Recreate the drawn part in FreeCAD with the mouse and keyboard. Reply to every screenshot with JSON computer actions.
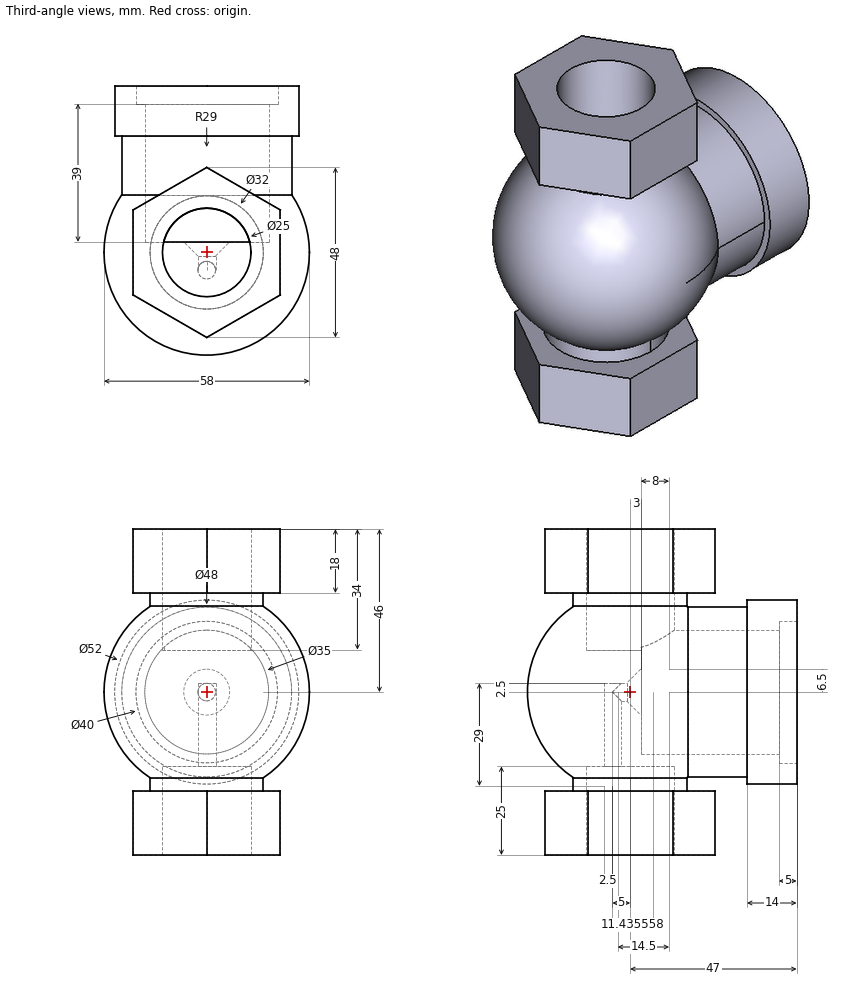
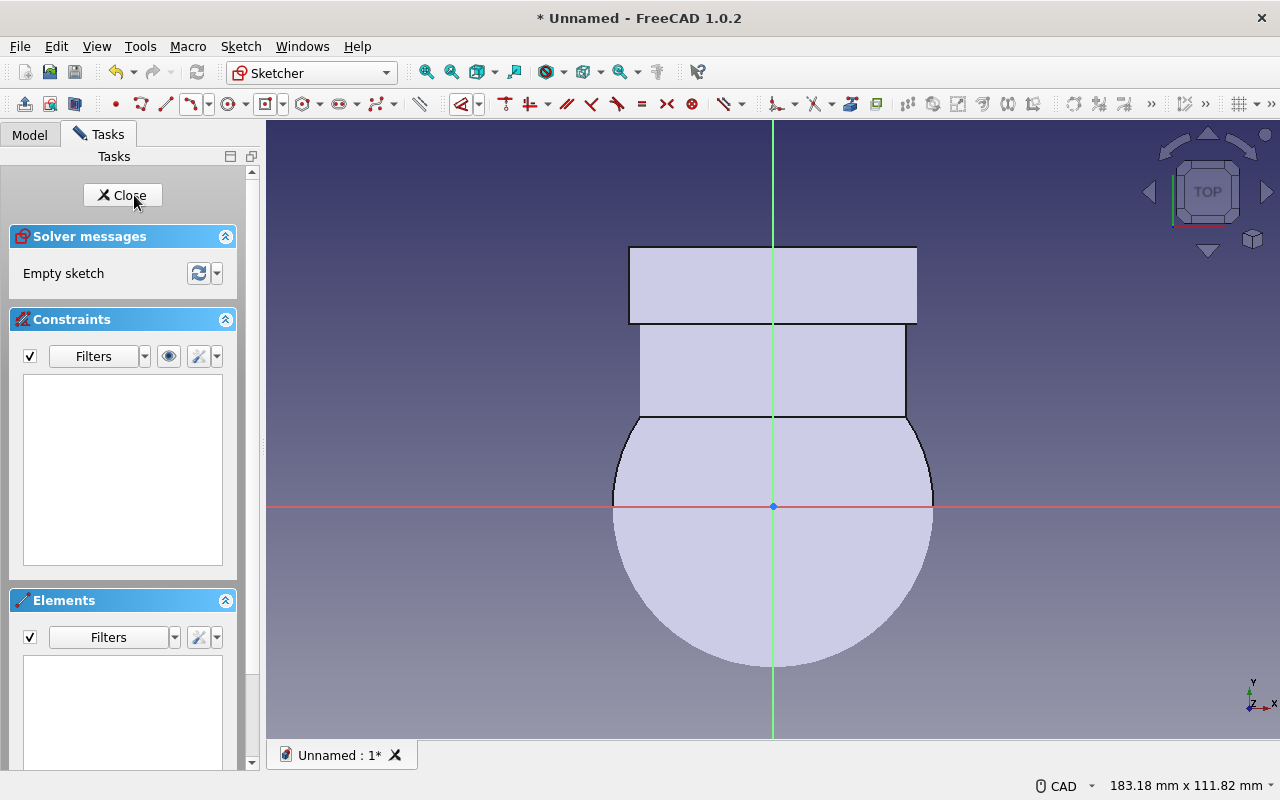
{"action": "scroll", "coordinate": [829, 570], "scroll_direction": "up", "scroll_amount": 4}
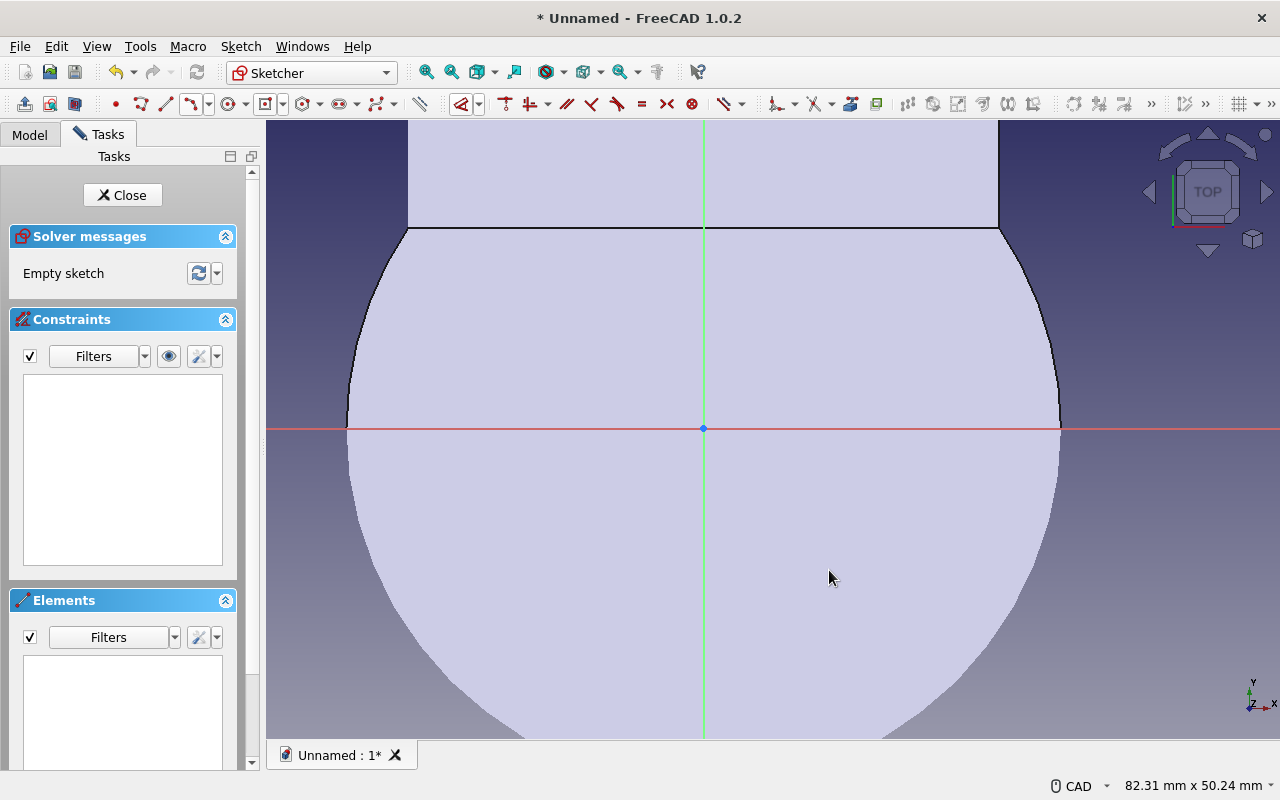
{"action": "key", "text": "g c"}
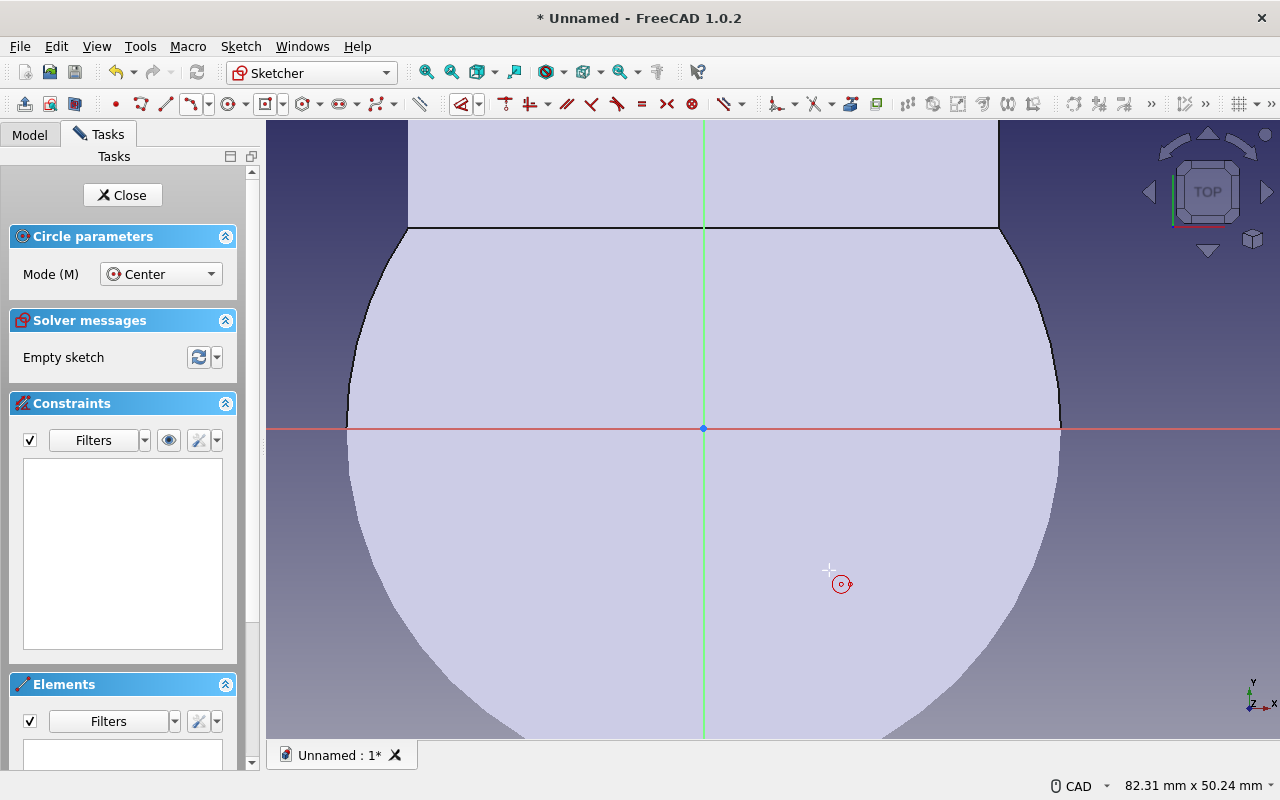
{"action": "left_click", "coordinate": [704, 429]}
{"action": "left_click", "coordinate": [843, 290]}
{"action": "key", "text": "Escape"}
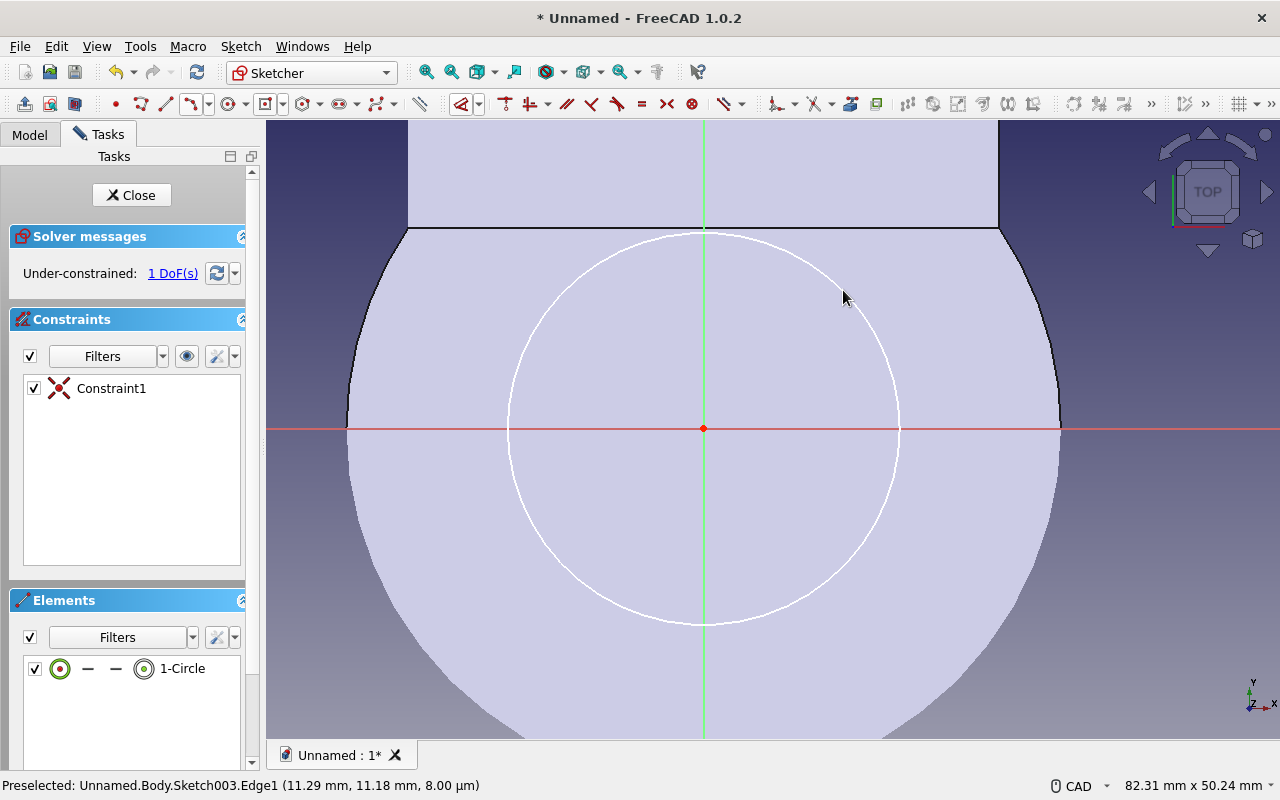
{"action": "left_click", "coordinate": [842, 290]}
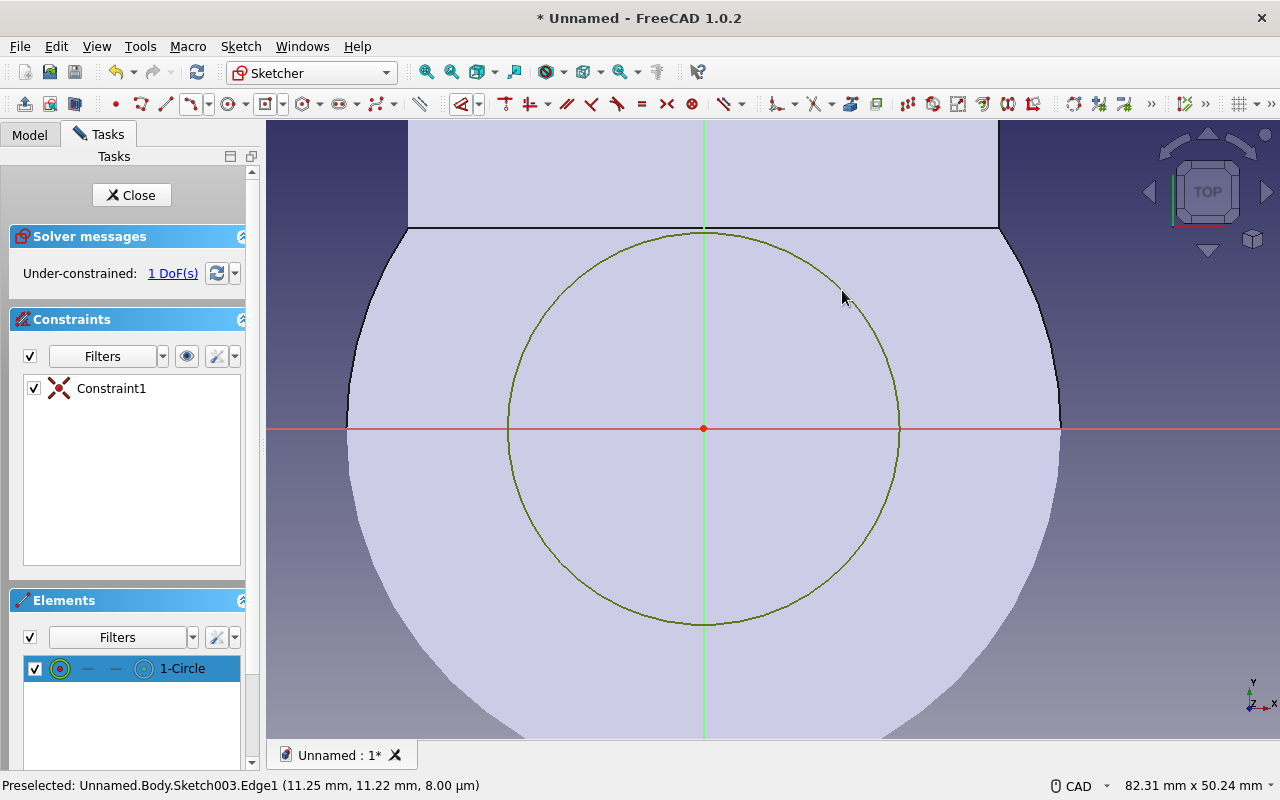
{"action": "key", "text": "k o"}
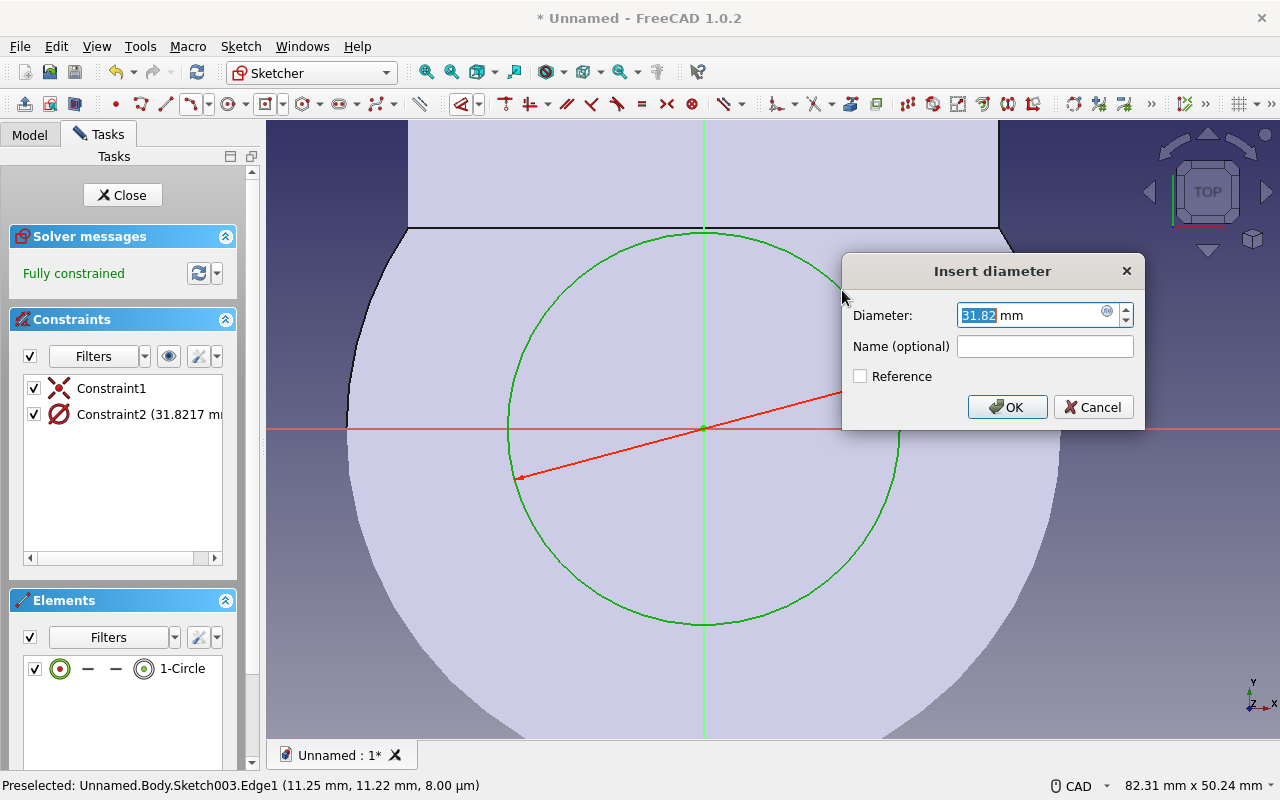
{"action": "type", "text": "32"}
{"action": "key", "text": "Return"}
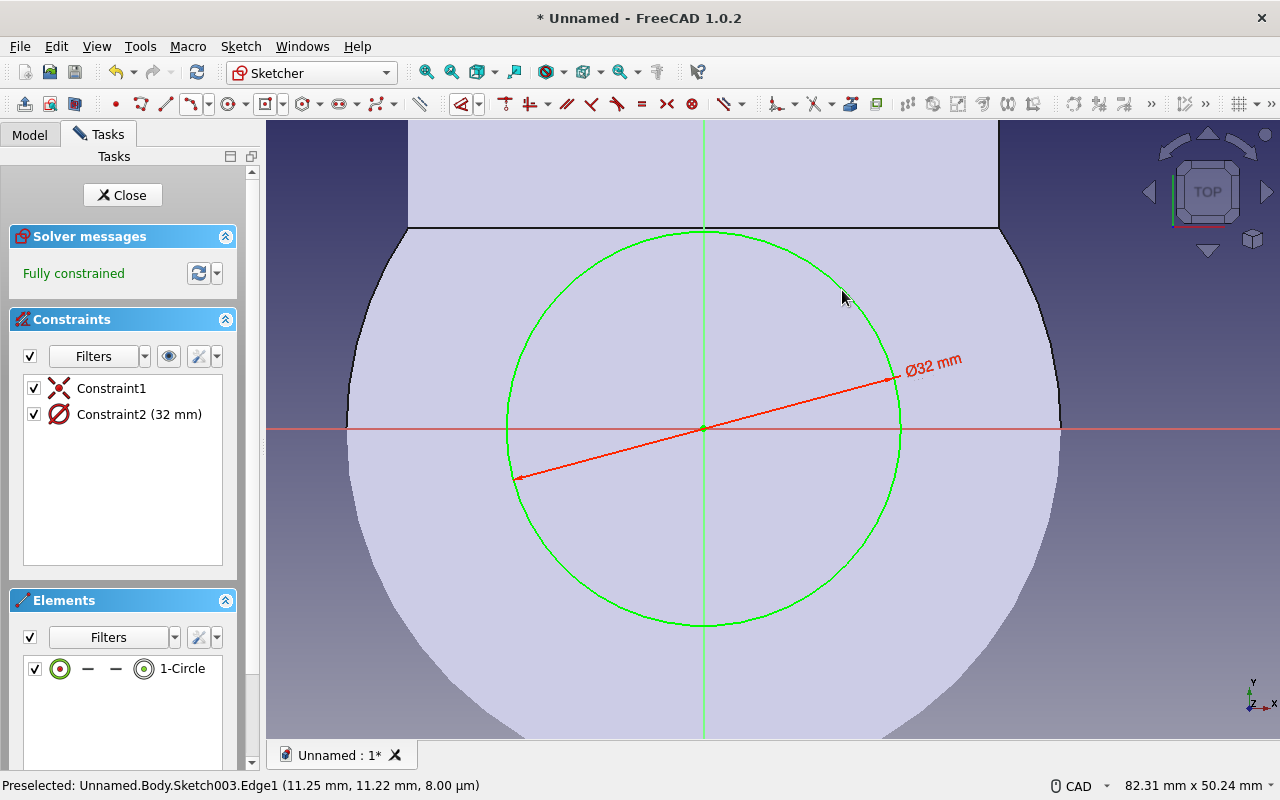
{"action": "left_click", "coordinate": [123, 195]}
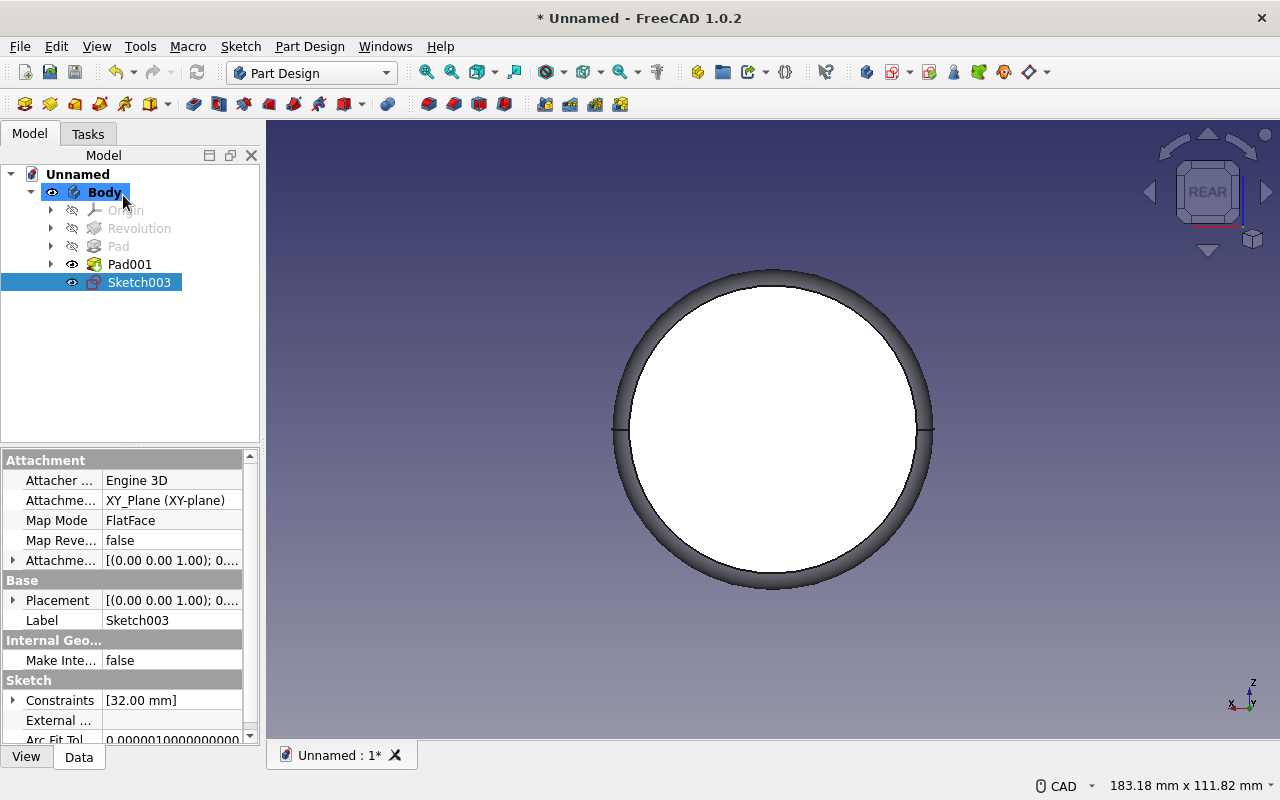
{"action": "left_click", "coordinate": [25, 104]}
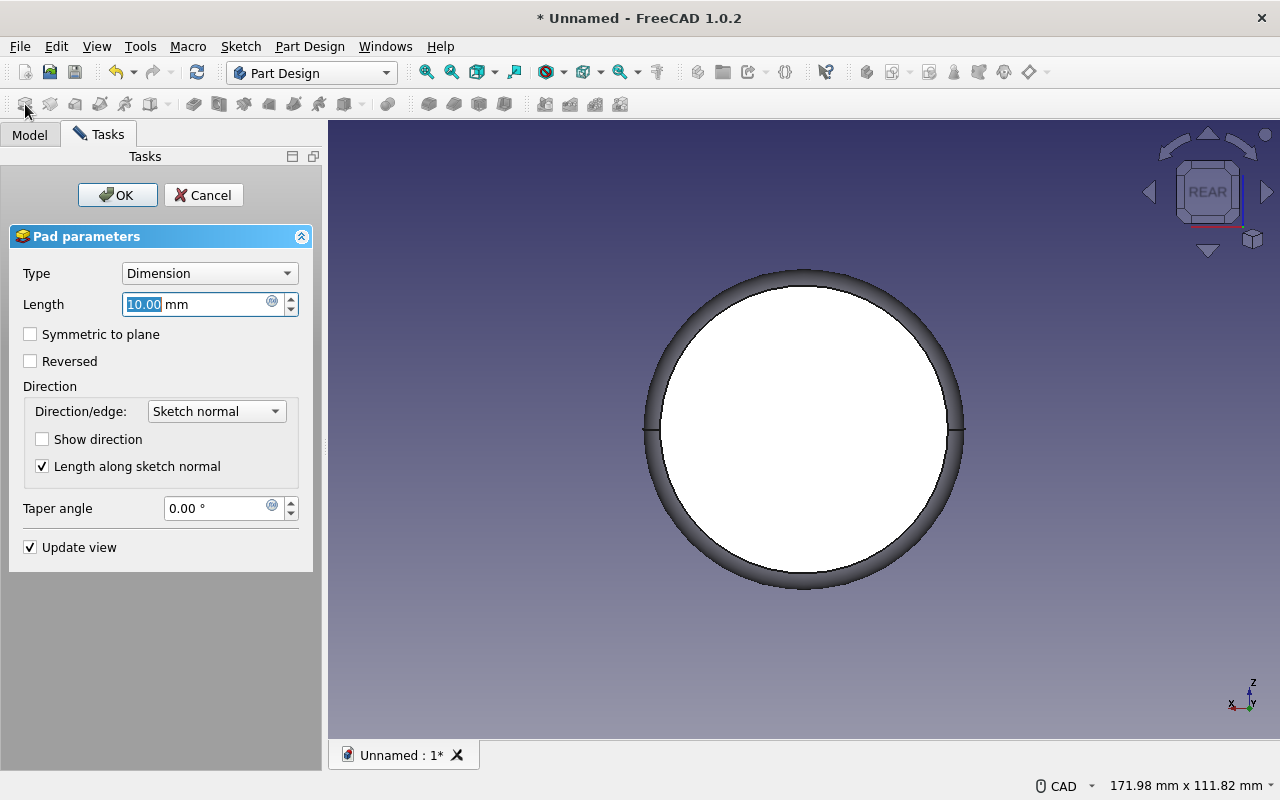
{"action": "type", "text": "46"}
{"action": "key", "text": "Tab"}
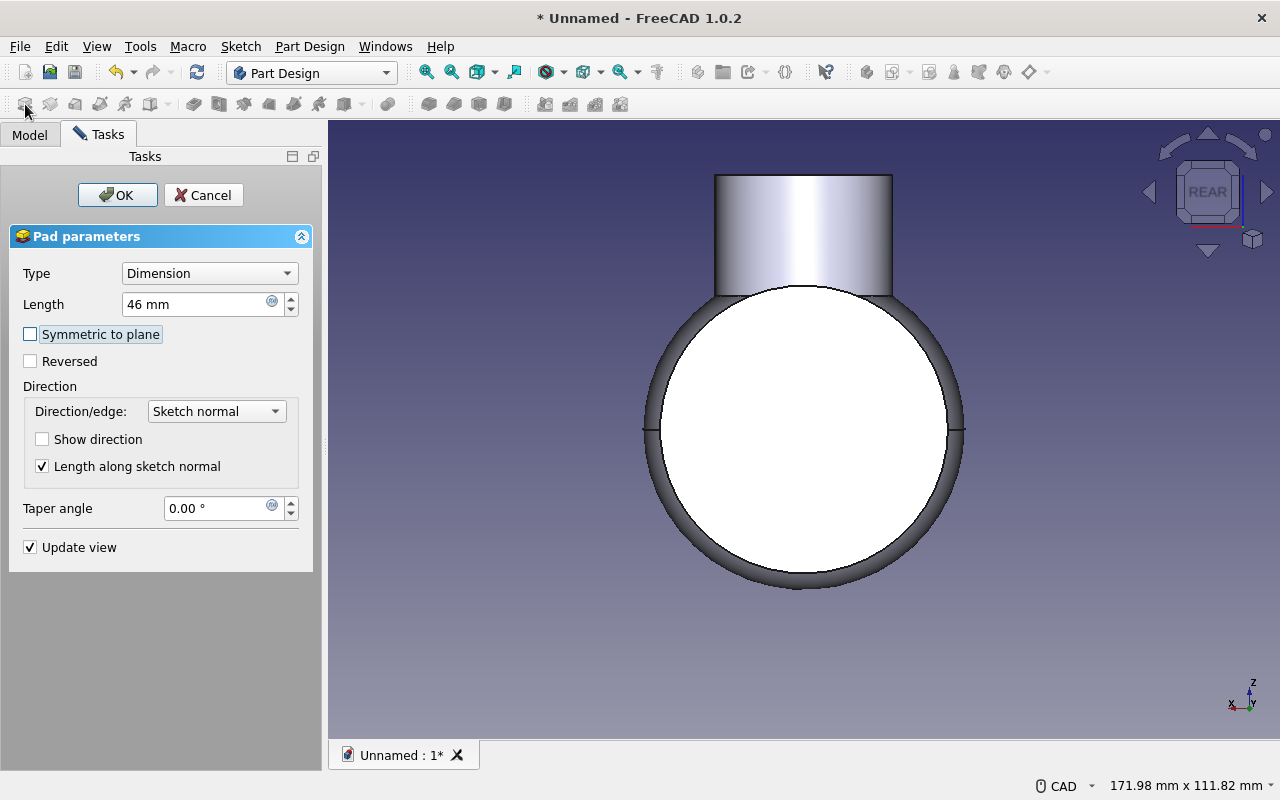
{"action": "left_click", "coordinate": [118, 195]}